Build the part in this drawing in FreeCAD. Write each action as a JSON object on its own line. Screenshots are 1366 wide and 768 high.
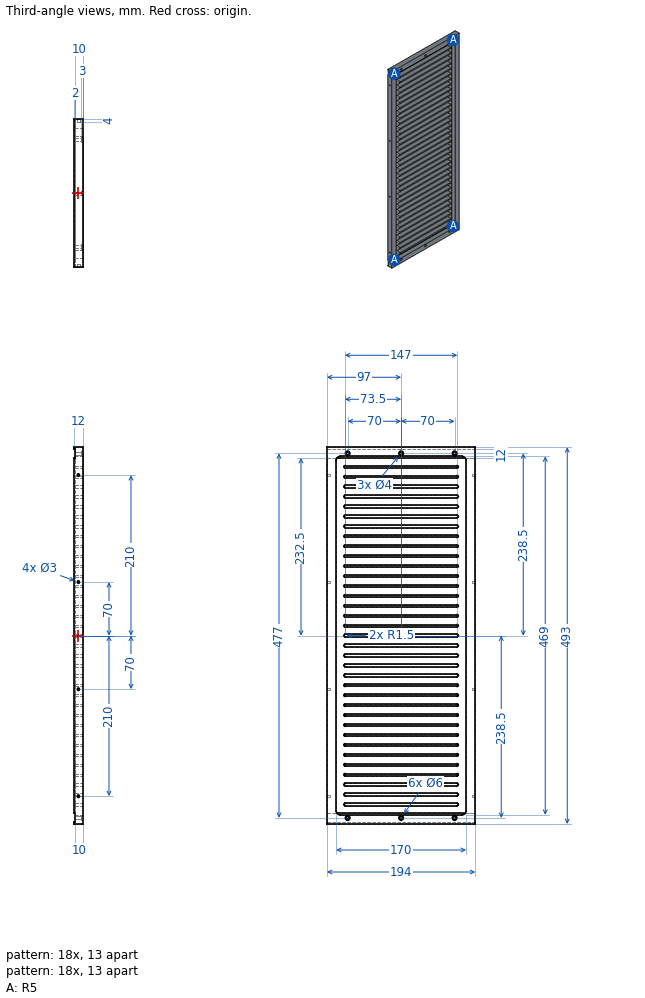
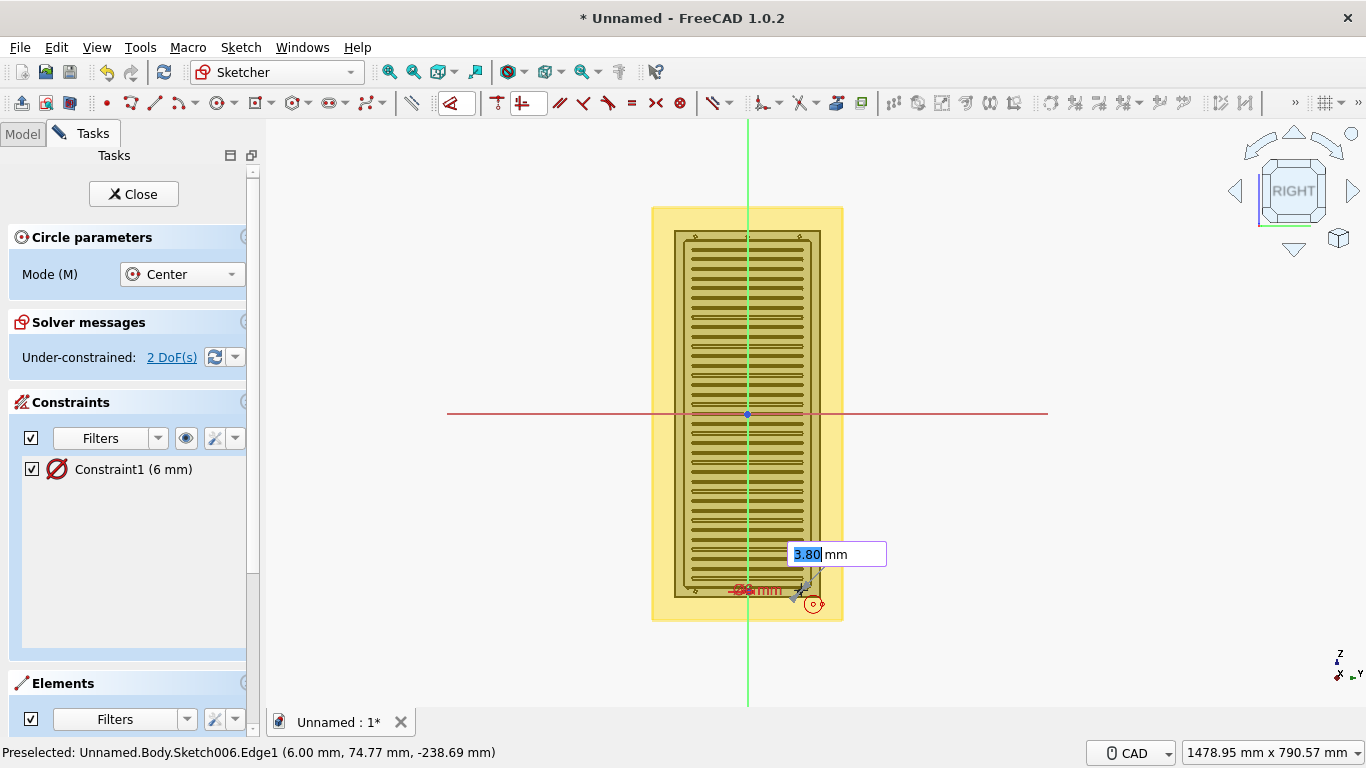
{"action": "type", "text": "6"}
{"action": "key", "text": "Return"}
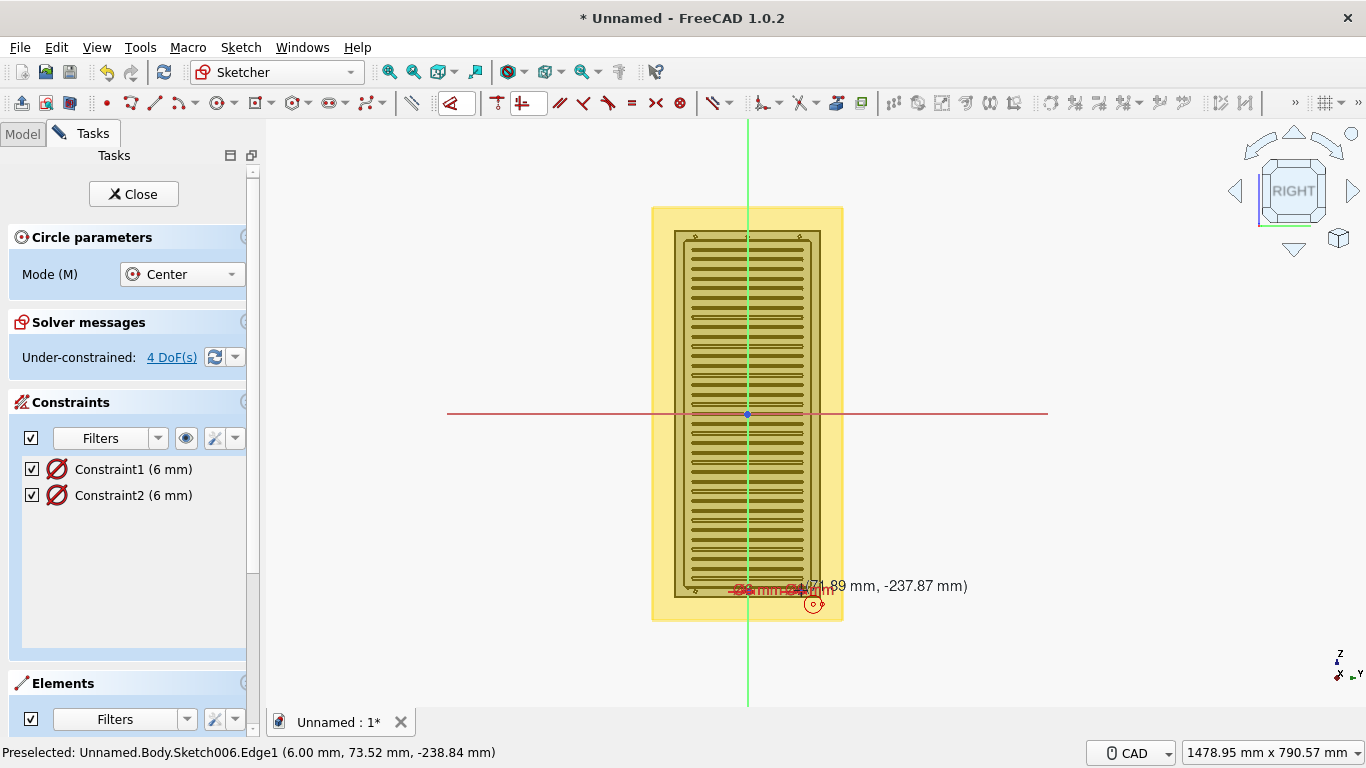
{"action": "scroll", "coordinate": [695, 591], "scroll_direction": "up", "scroll_amount": 12}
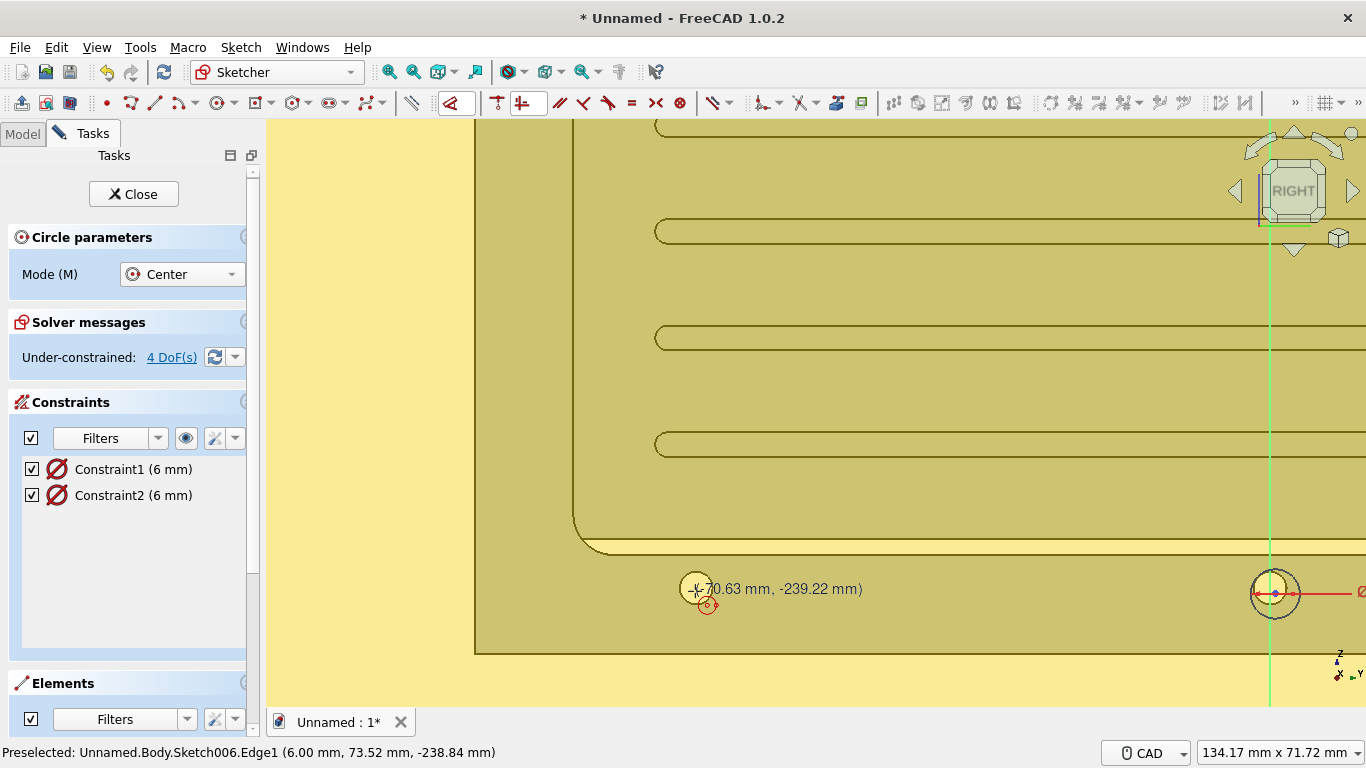
{"action": "scroll", "coordinate": [695, 591], "scroll_direction": "down", "scroll_amount": 12}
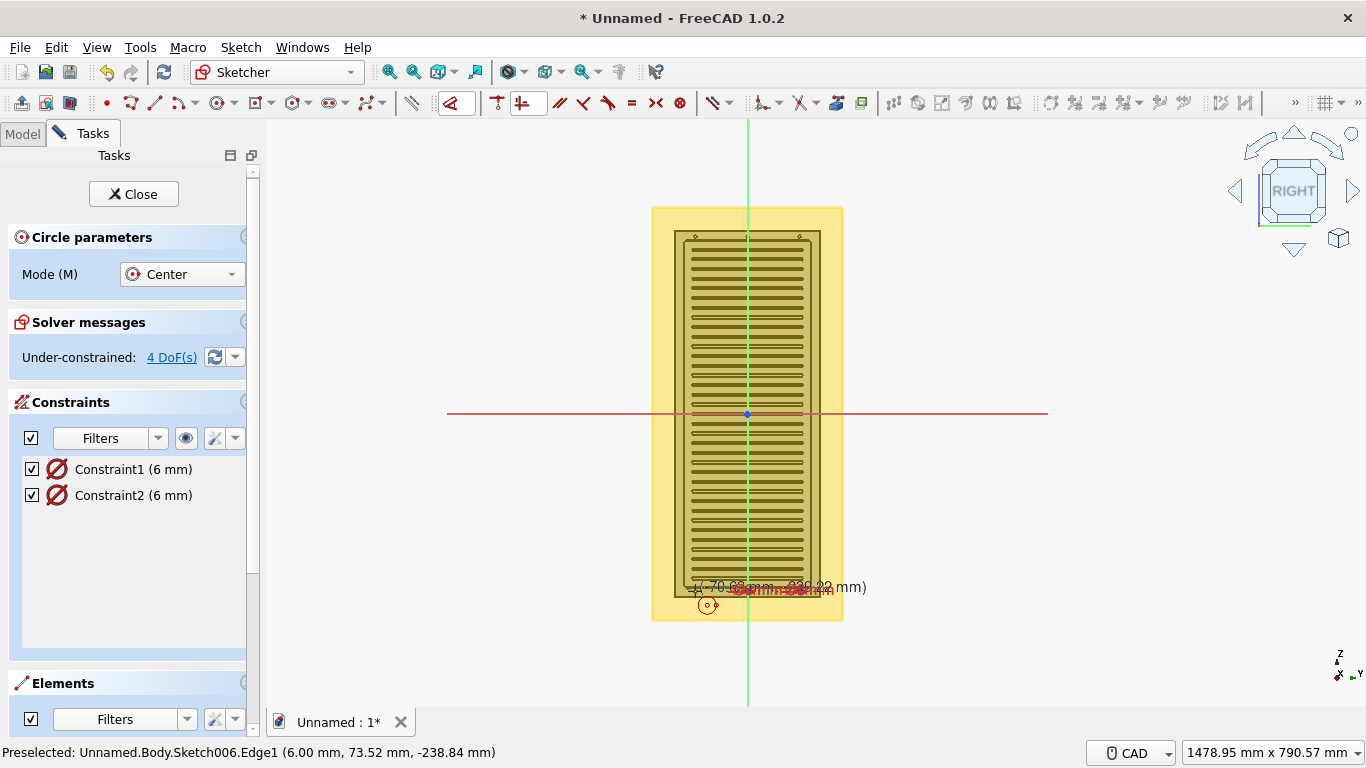
{"action": "left_click", "coordinate": [695, 591]}
{"action": "mouse_move", "coordinate": [697, 590]}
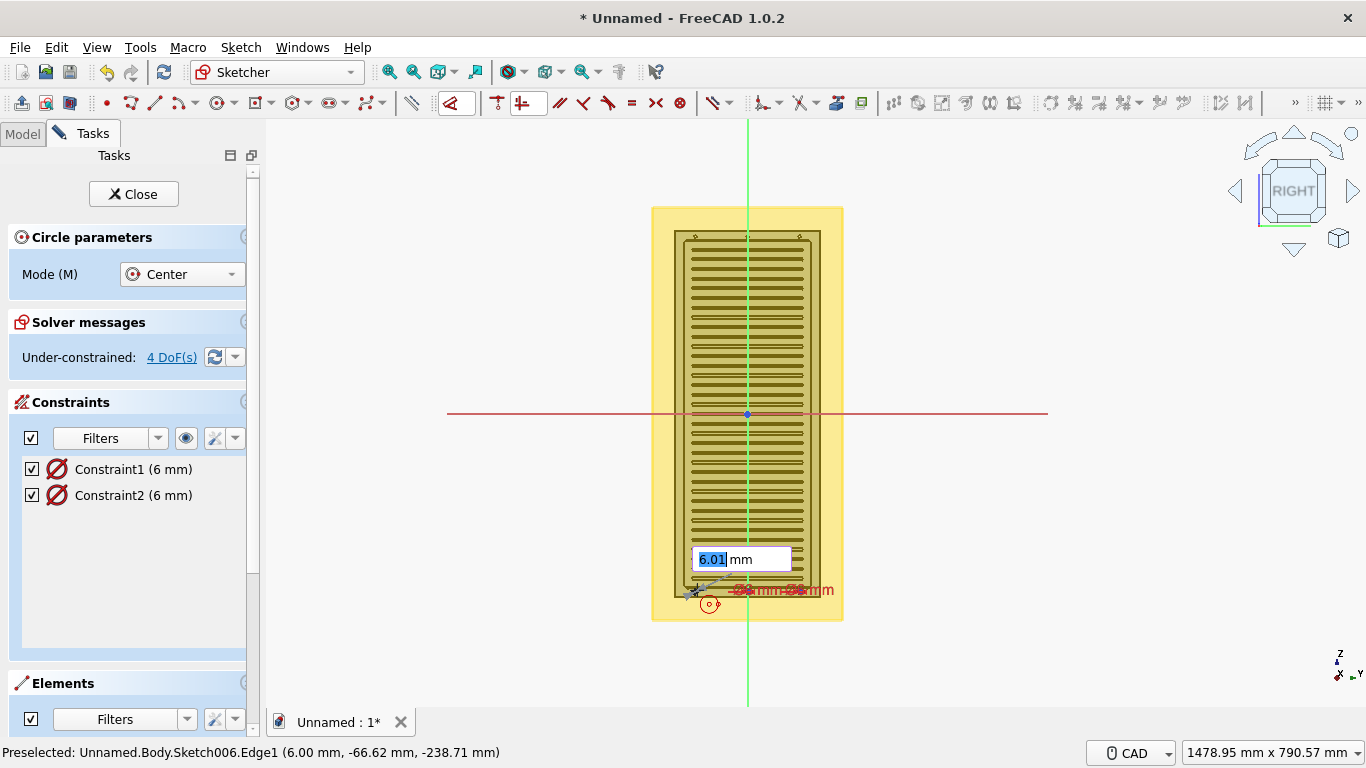
{"action": "type", "text": "6"}
{"action": "key", "text": "Return"}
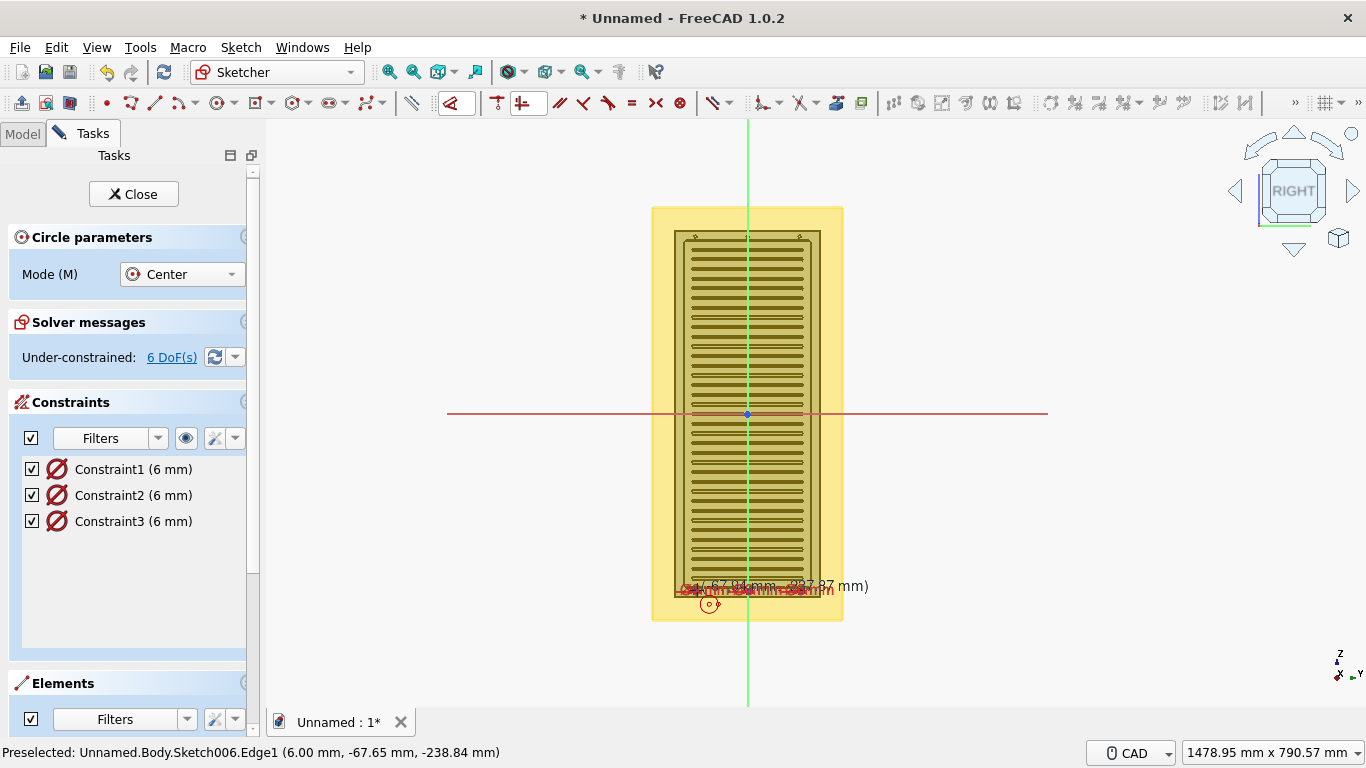
{"action": "scroll", "coordinate": [695, 237], "scroll_direction": "up", "scroll_amount": 12}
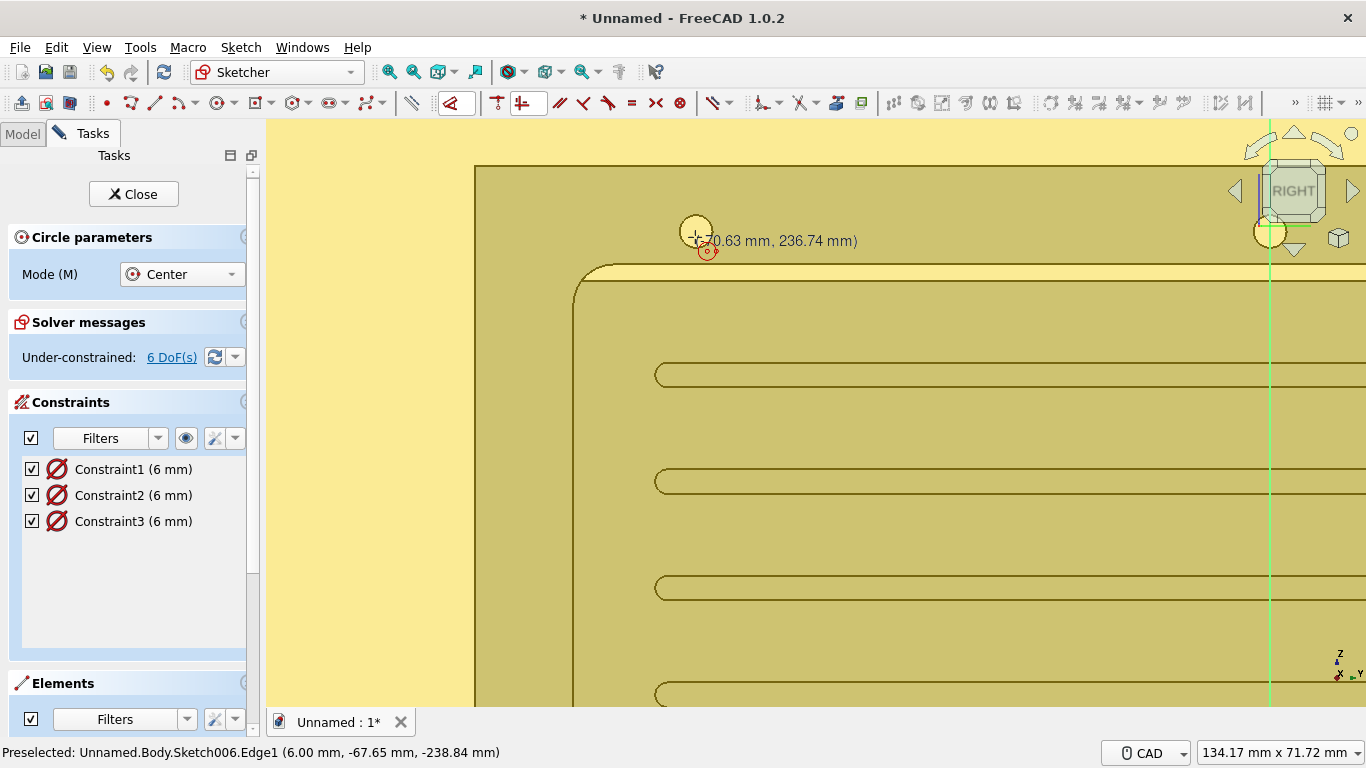
{"action": "scroll", "coordinate": [695, 236], "scroll_direction": "down", "scroll_amount": 12}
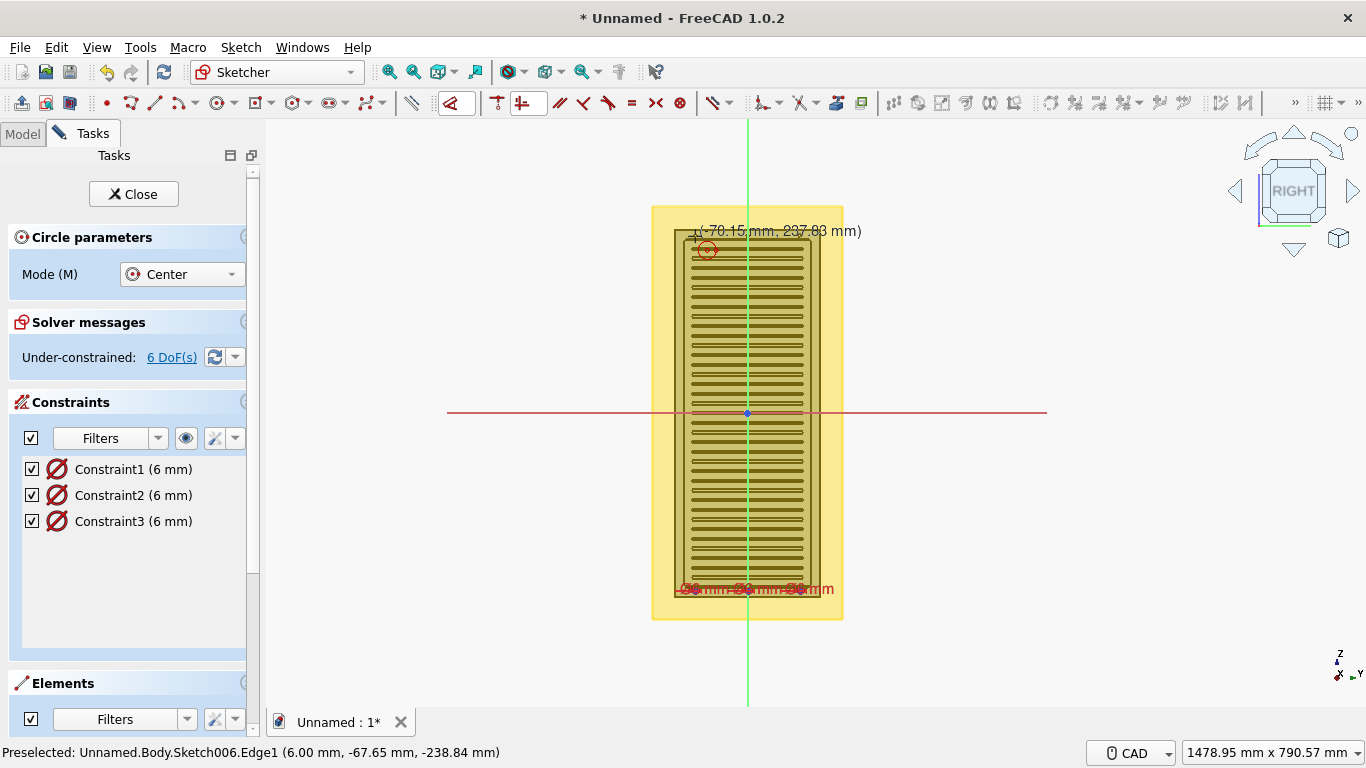
{"action": "left_click", "coordinate": [695, 236]}
{"action": "mouse_move", "coordinate": [697, 234]}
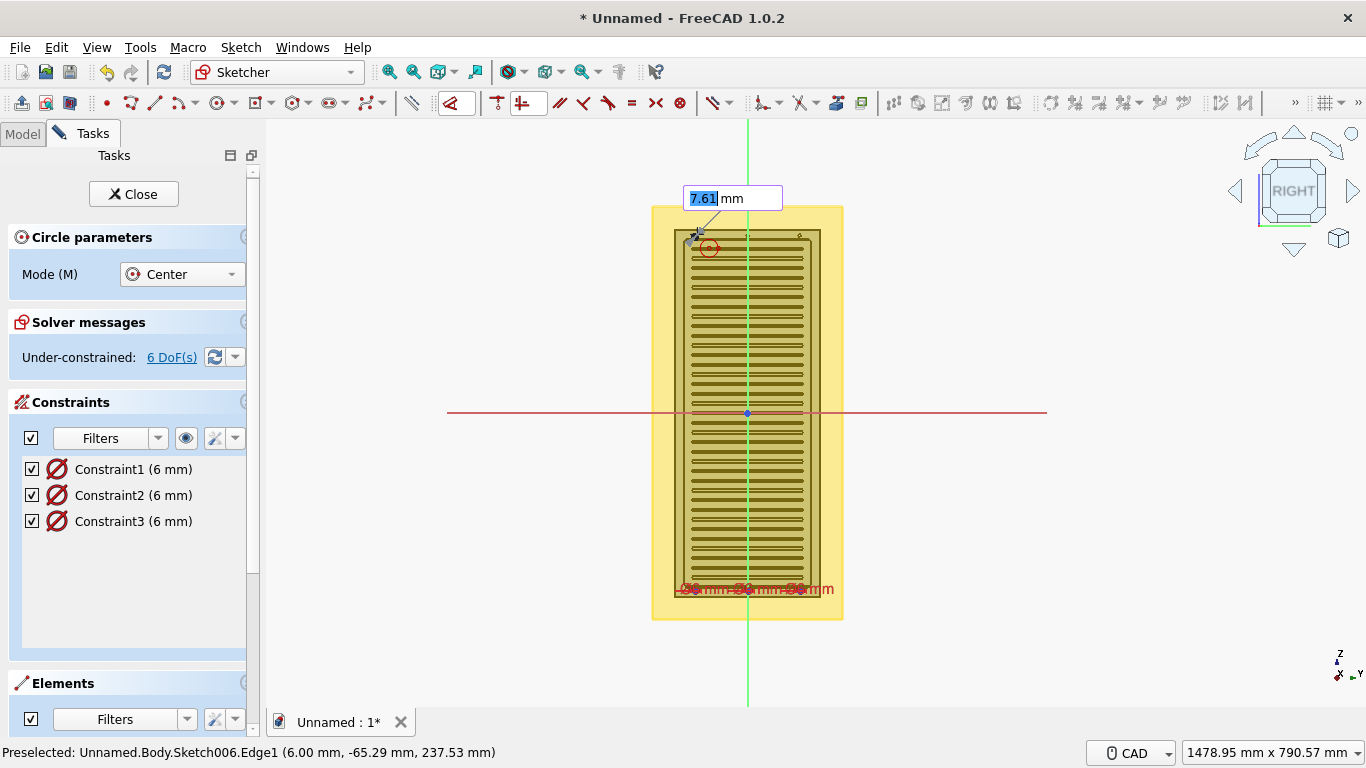
{"action": "type", "text": "6"}
{"action": "key", "text": "Return"}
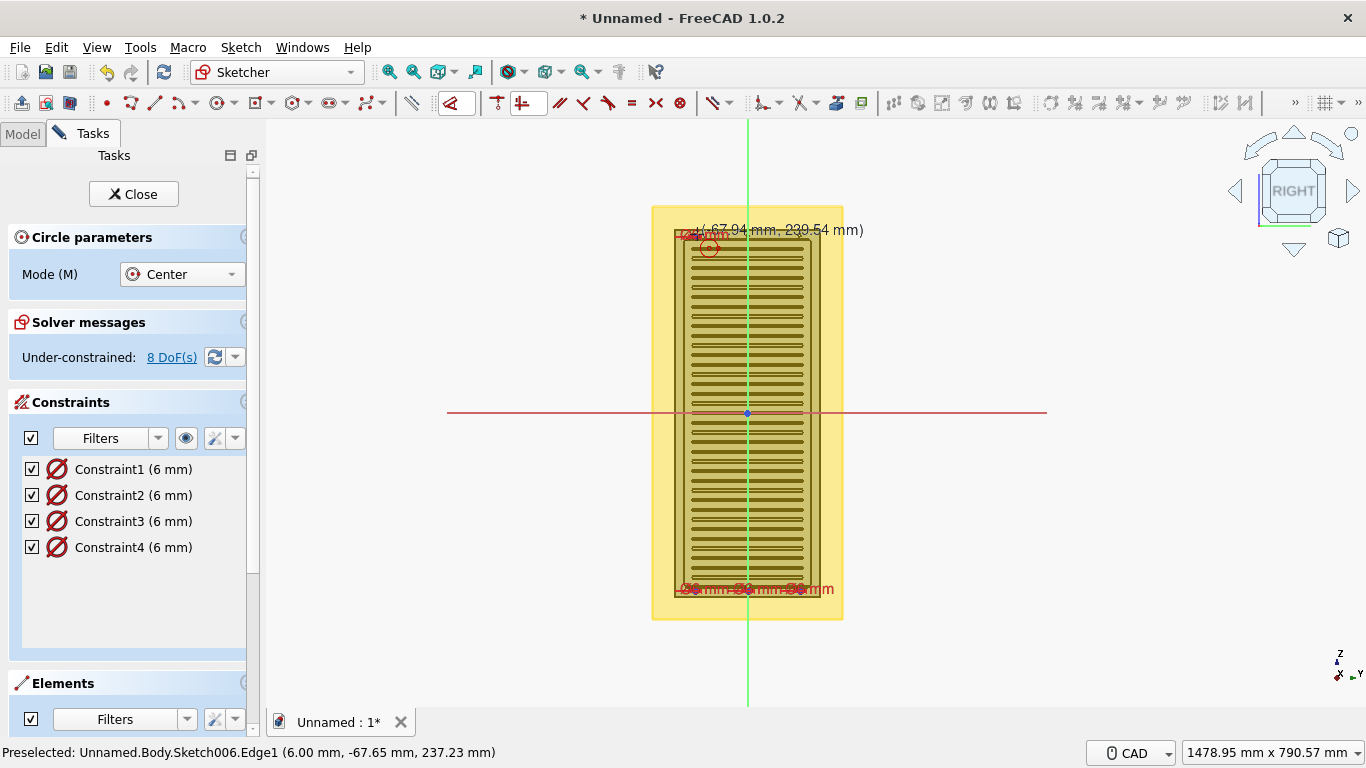
{"action": "scroll", "coordinate": [748, 236], "scroll_direction": "up", "scroll_amount": 12}